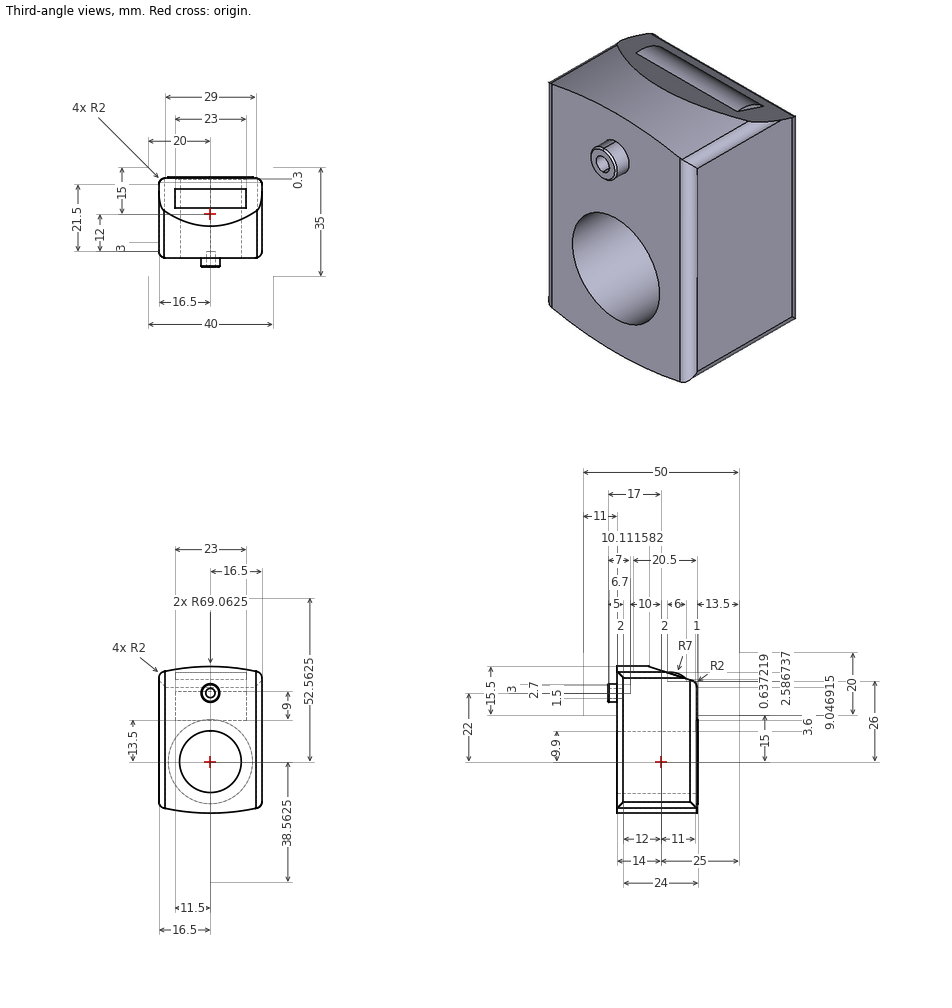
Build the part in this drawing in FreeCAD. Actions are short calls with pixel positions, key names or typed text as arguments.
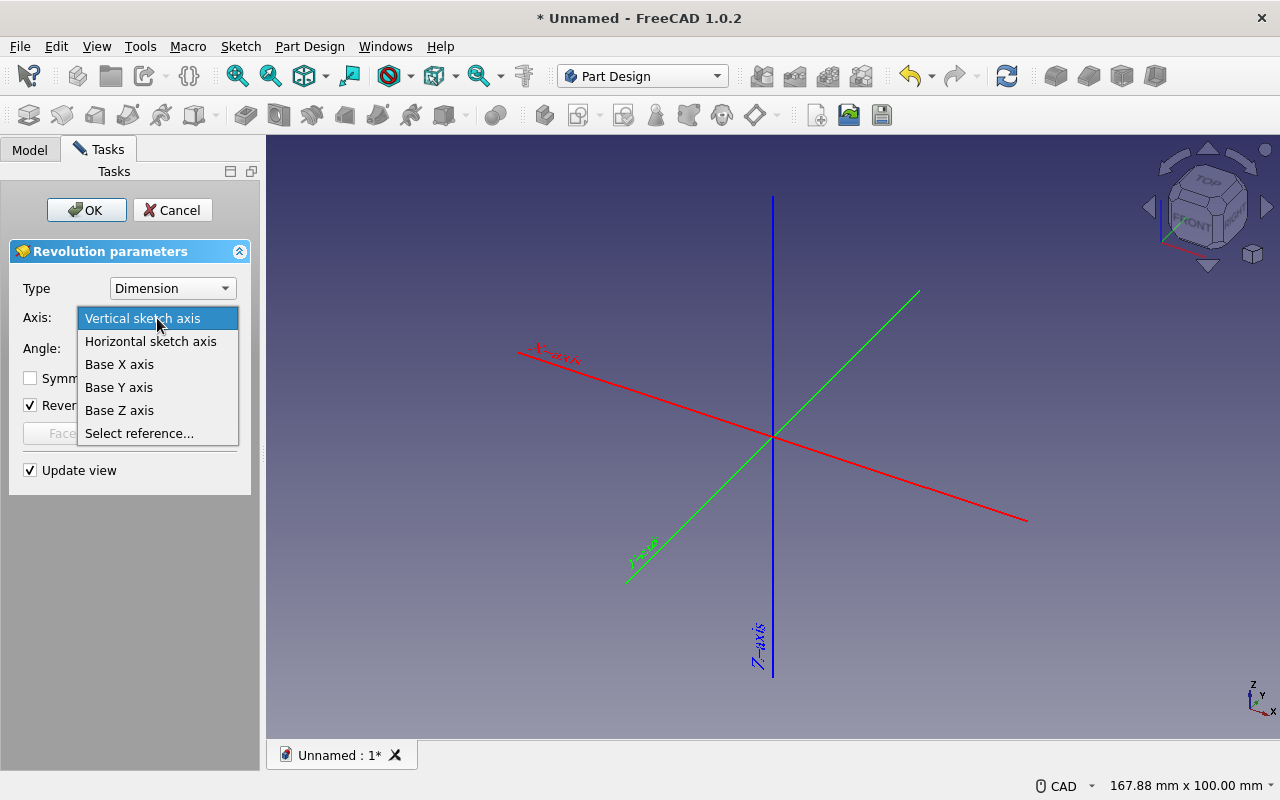
click(156, 342)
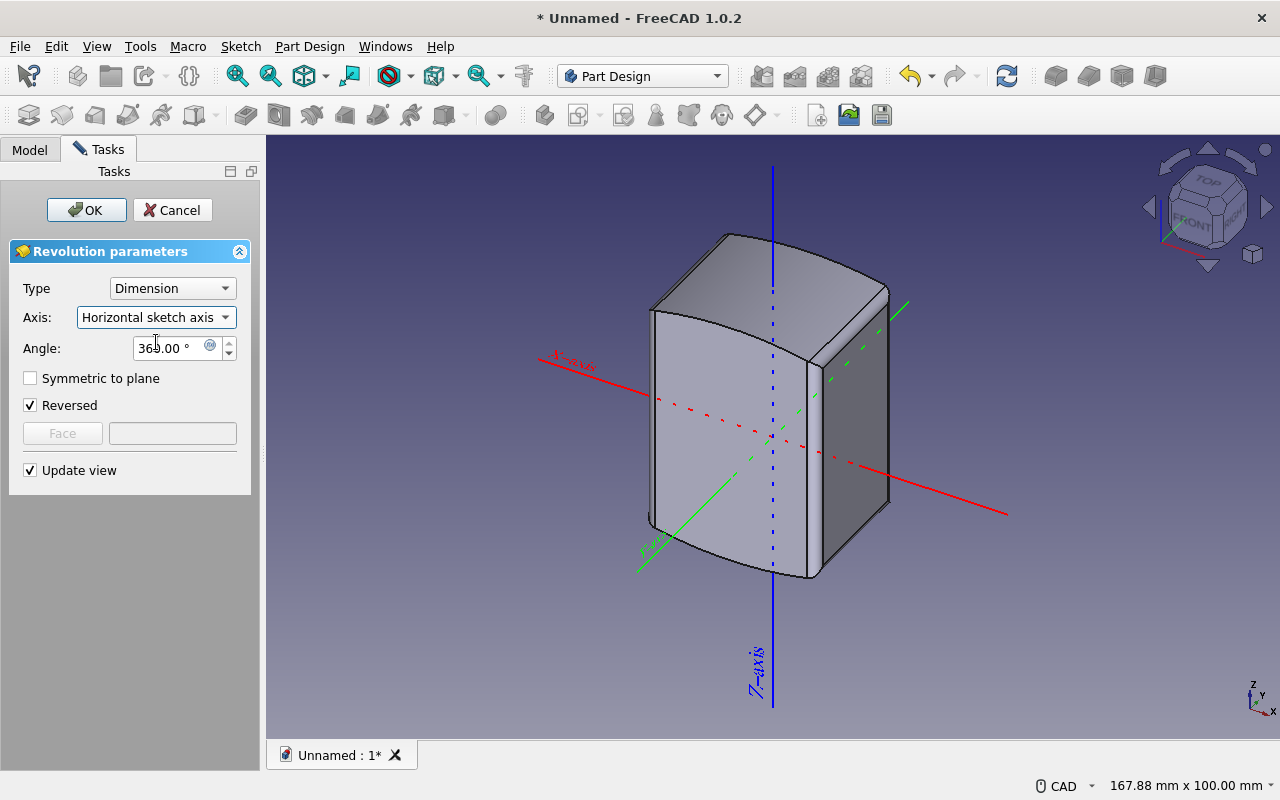
click(87, 210)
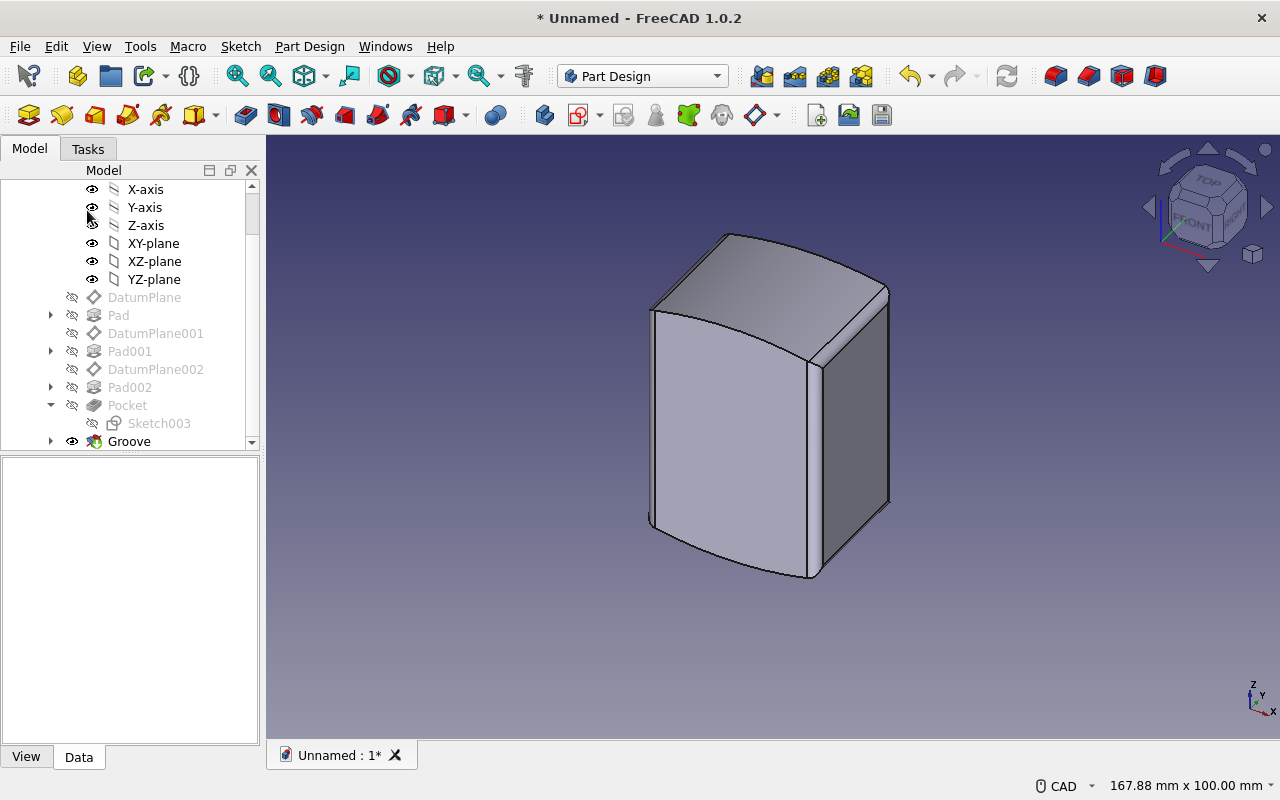
click(578, 116)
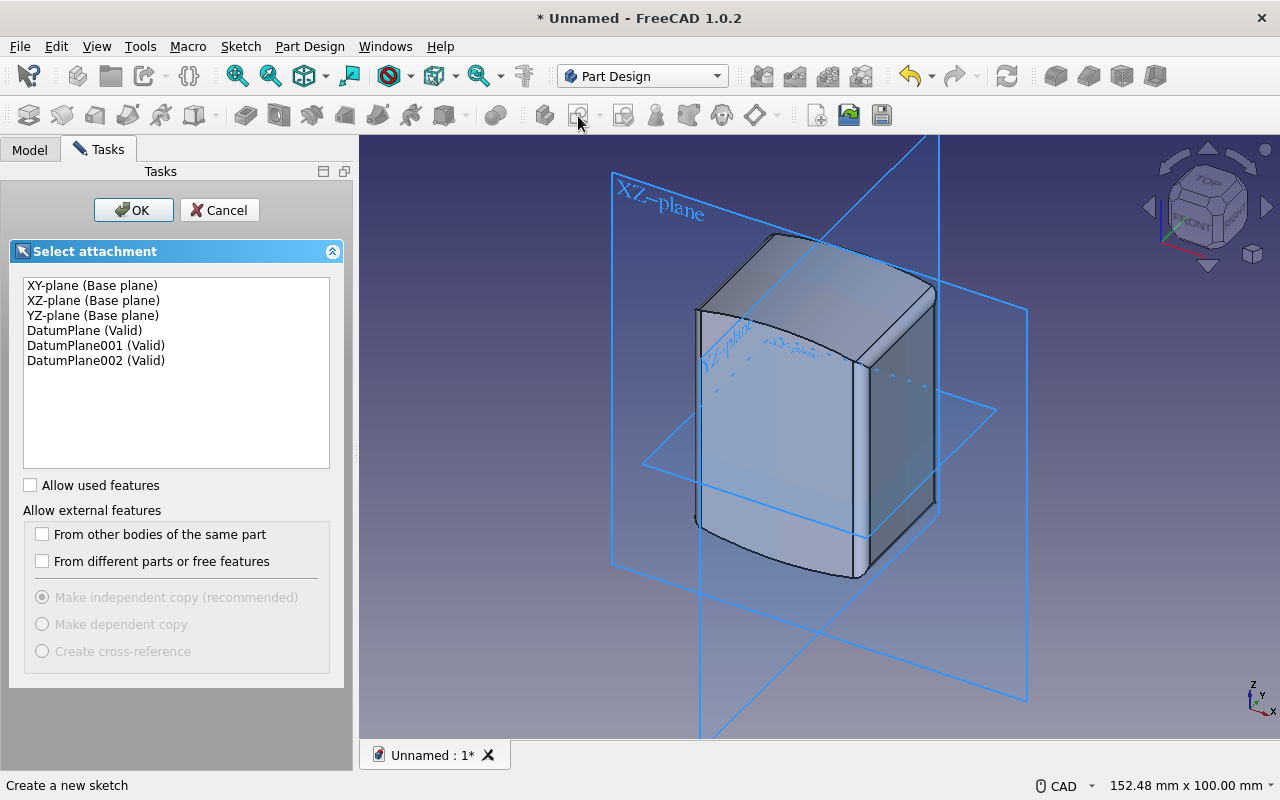
click(84, 316)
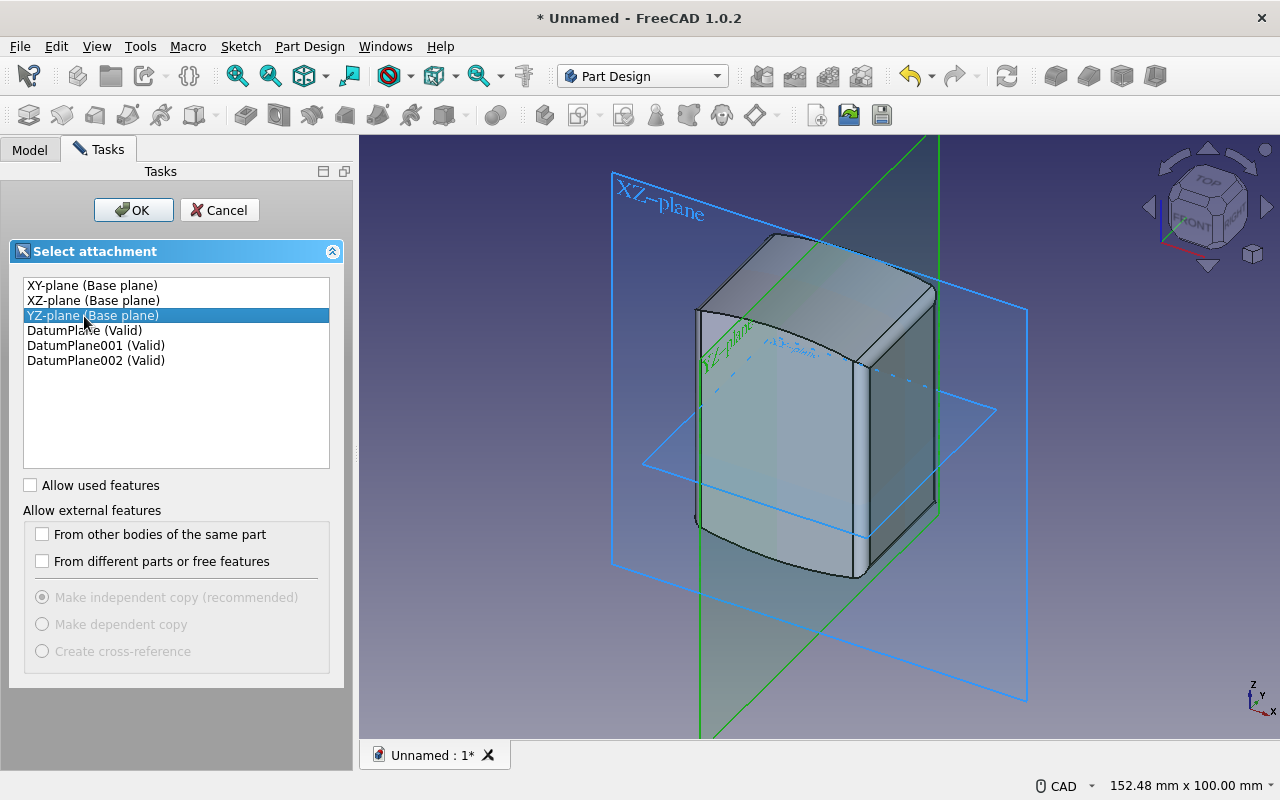
click(134, 210)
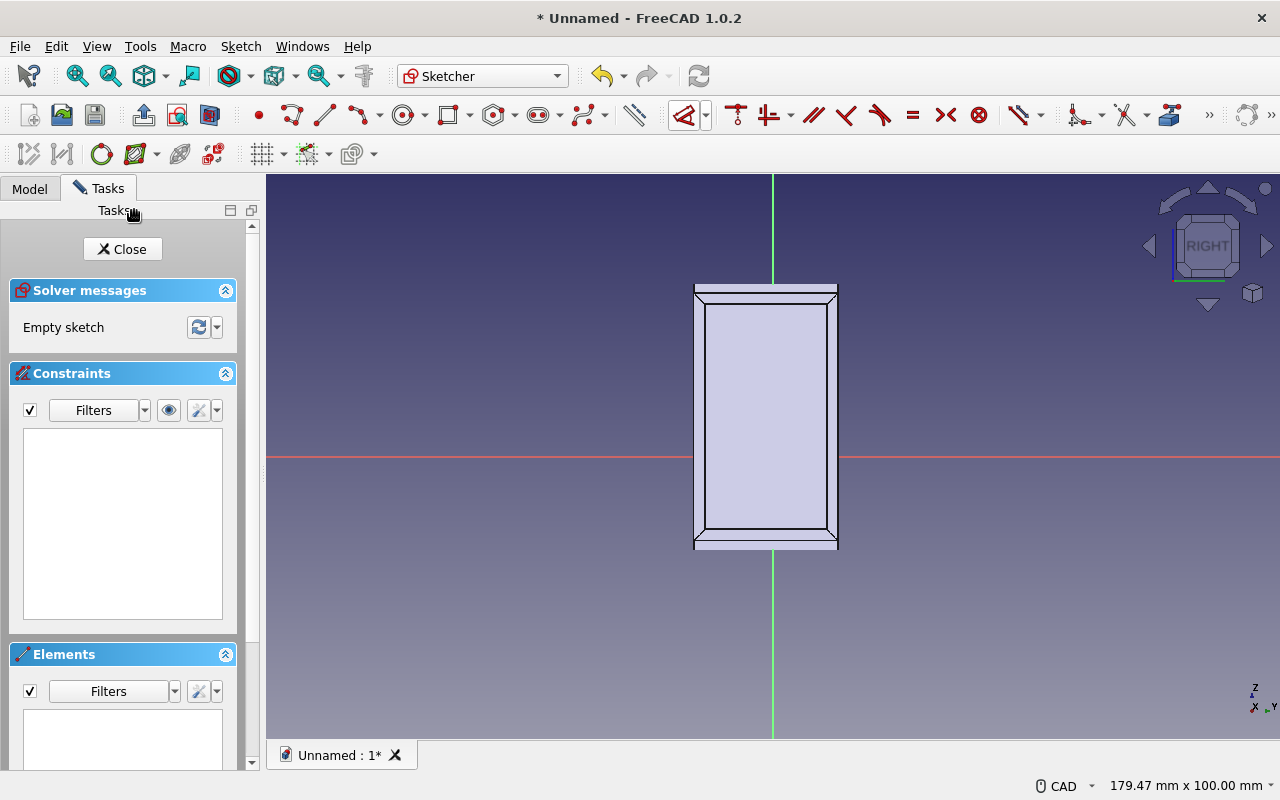
click(210, 116)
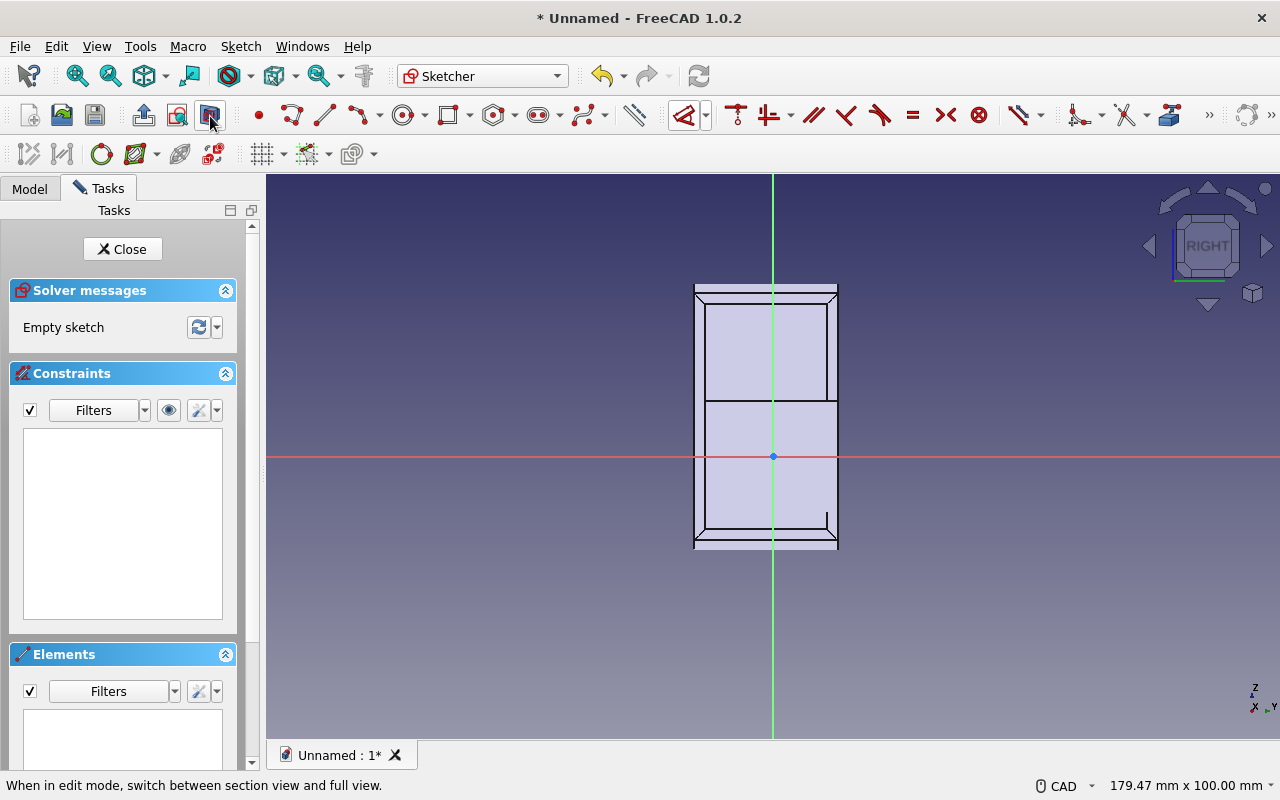
scroll(739, 423, up, 9)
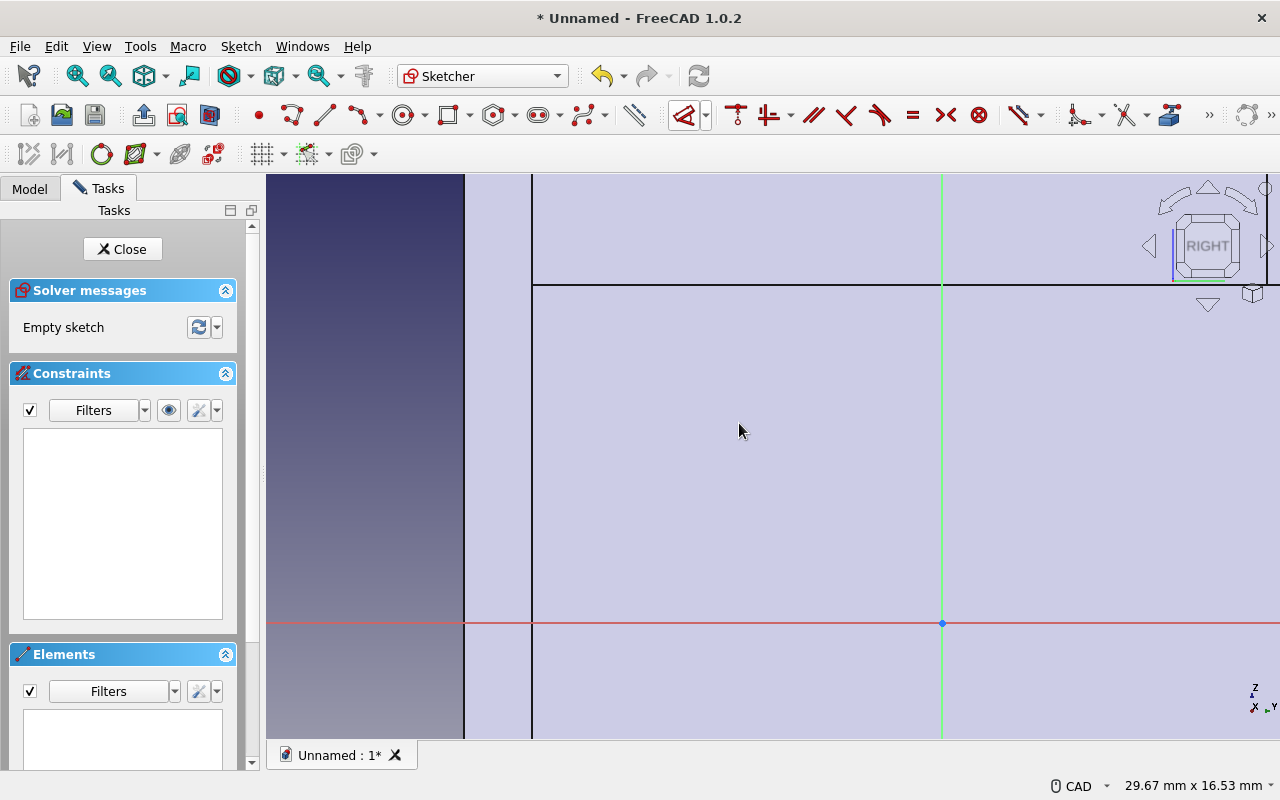
click(448, 116)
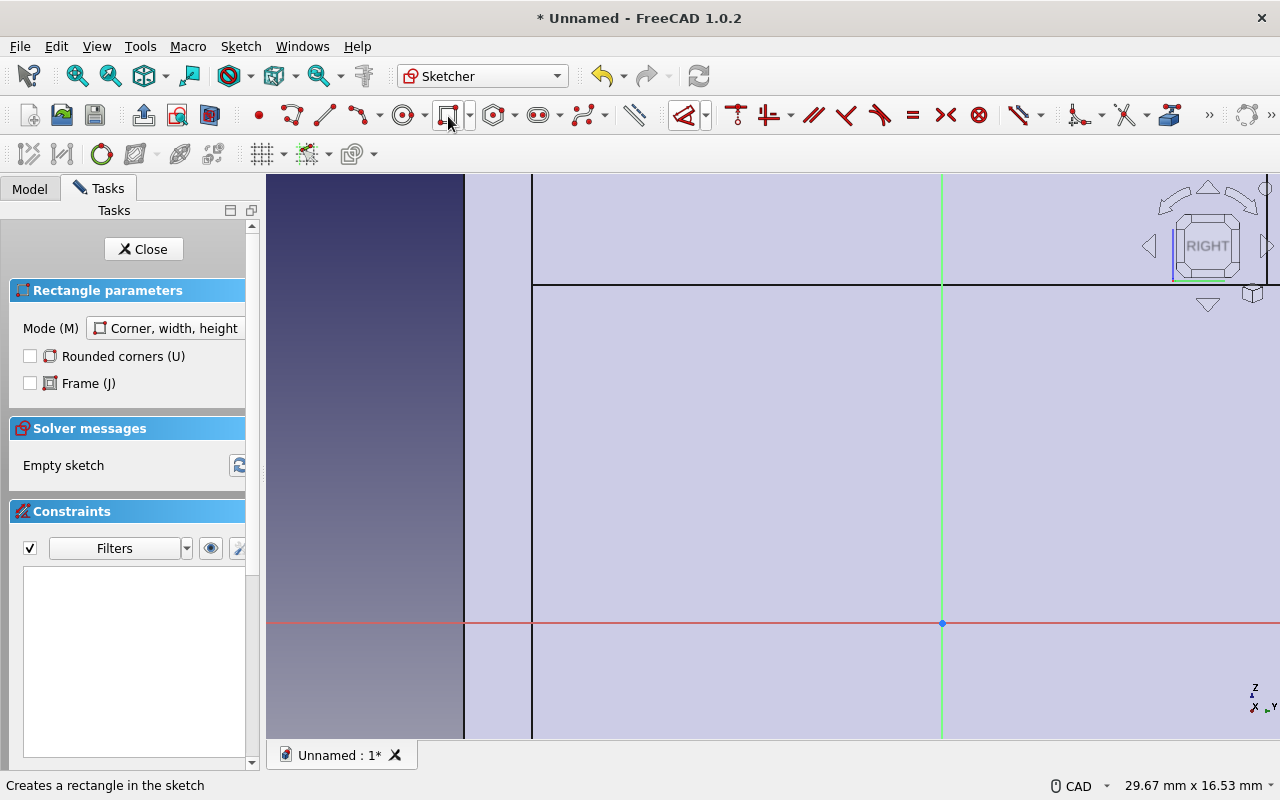
click(464, 285)
click(532, 623)
key(Escape)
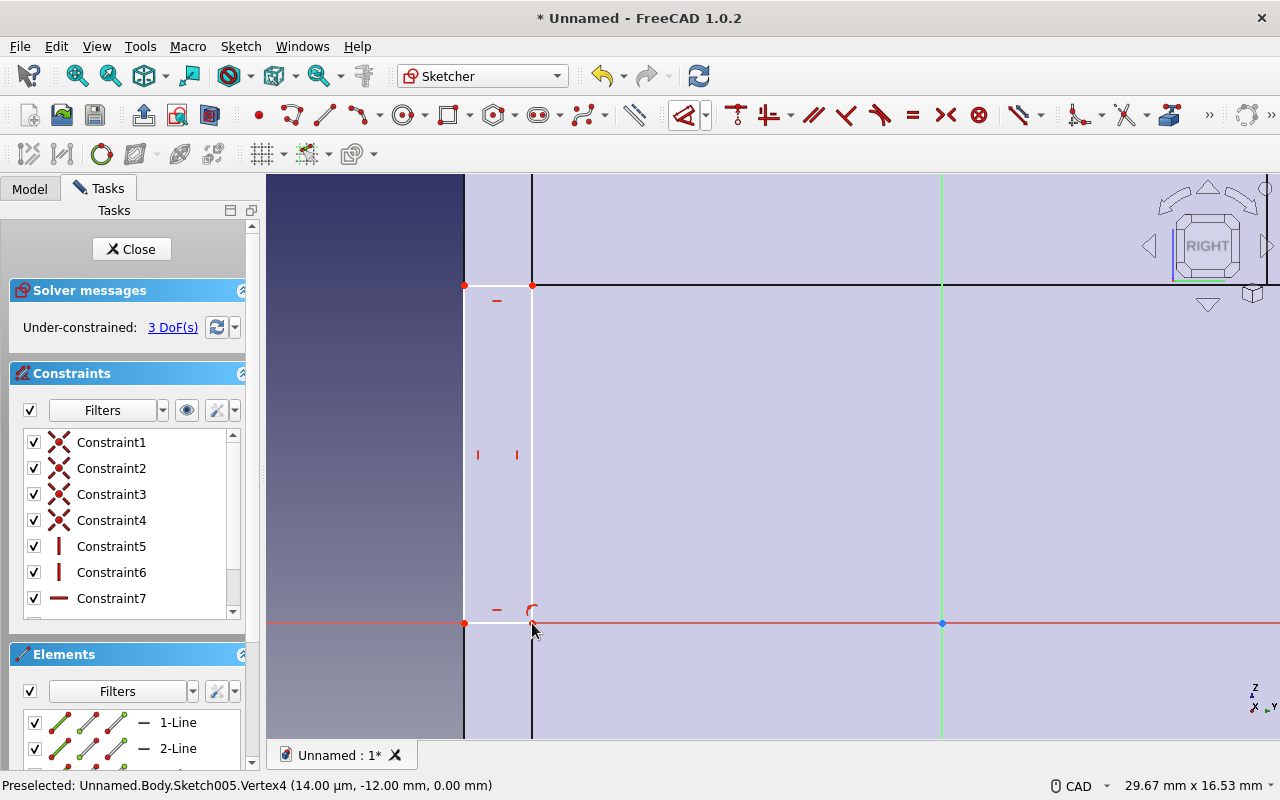
click(484, 623)